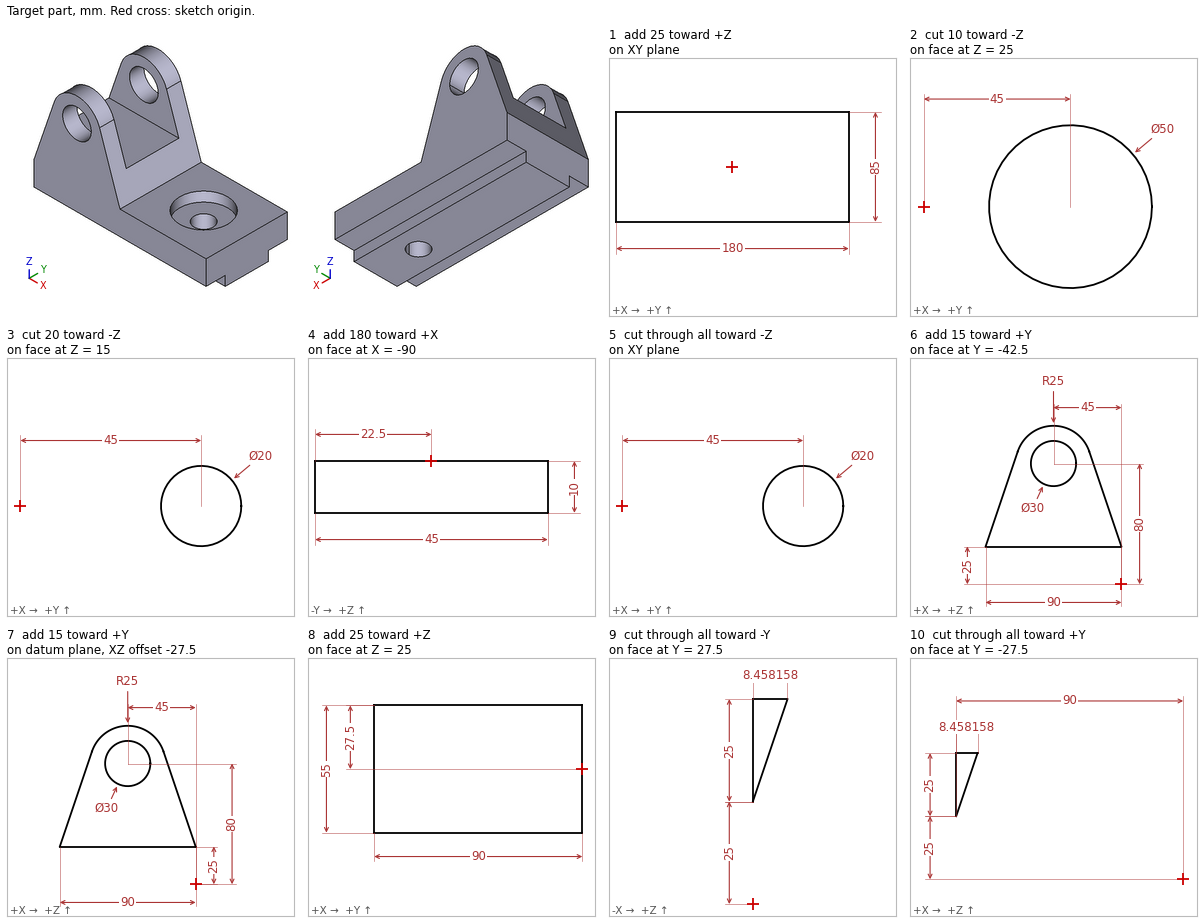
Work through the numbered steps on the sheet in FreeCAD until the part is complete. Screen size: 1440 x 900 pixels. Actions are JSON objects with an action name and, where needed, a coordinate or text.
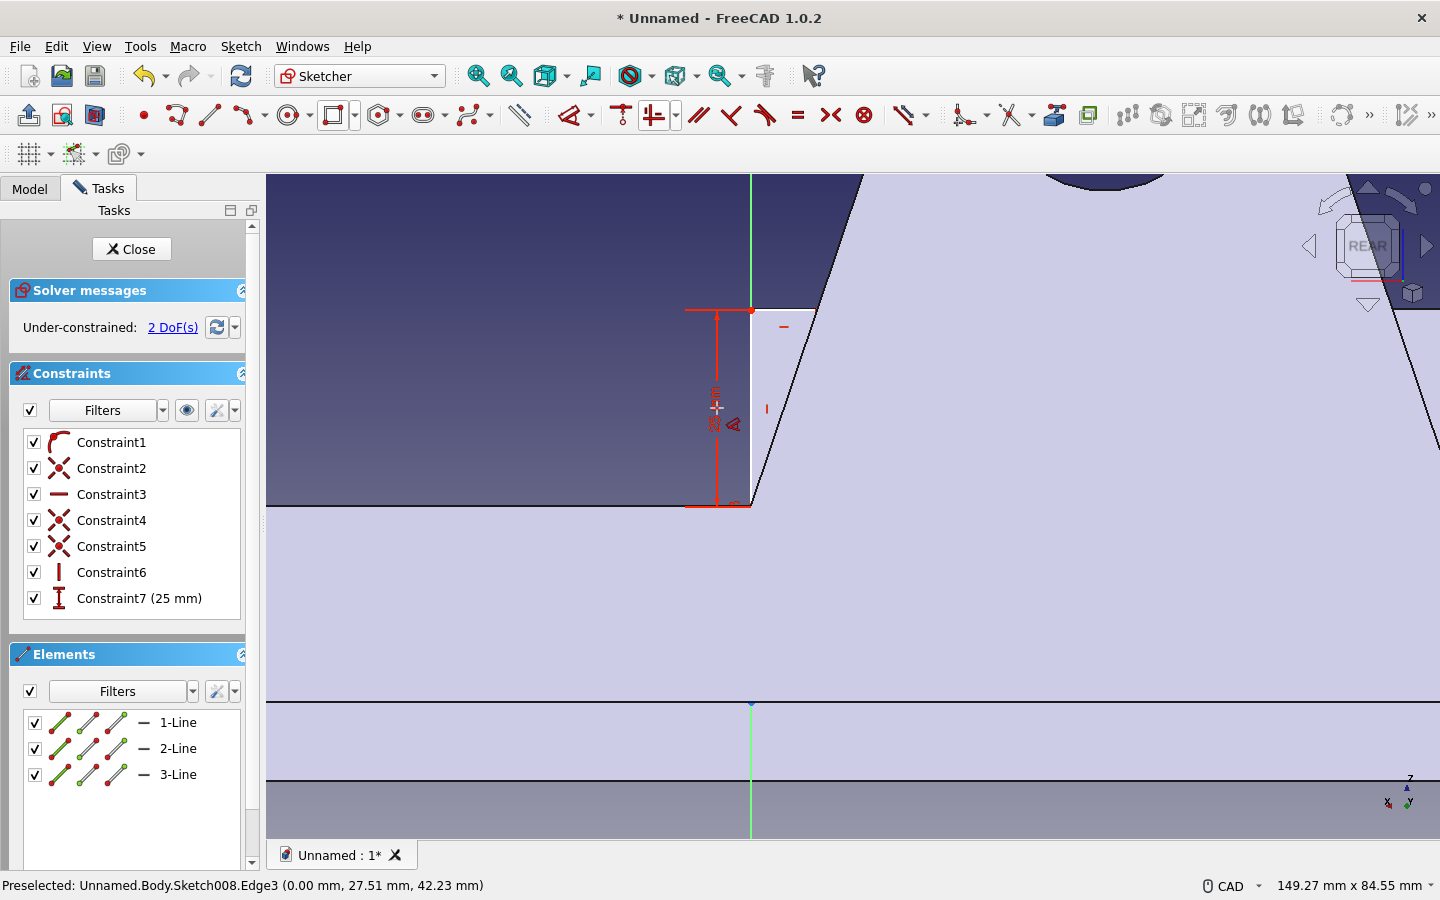
{"action": "left_click", "coordinate": [751, 507]}
{"action": "left_click", "coordinate": [717, 605]}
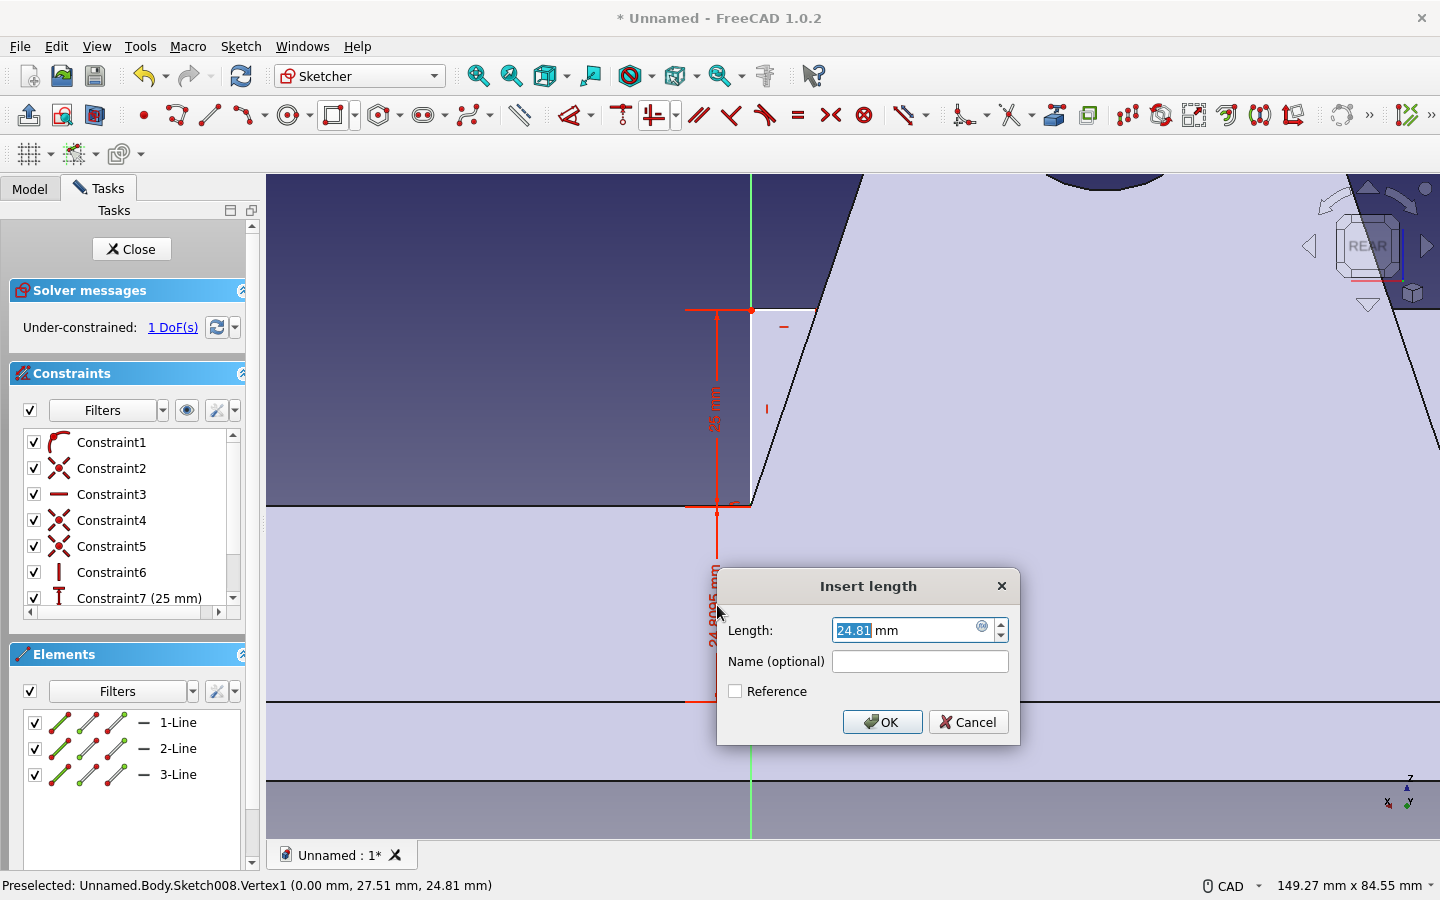
{"action": "type", "text": "25"}
{"action": "key", "text": "Return"}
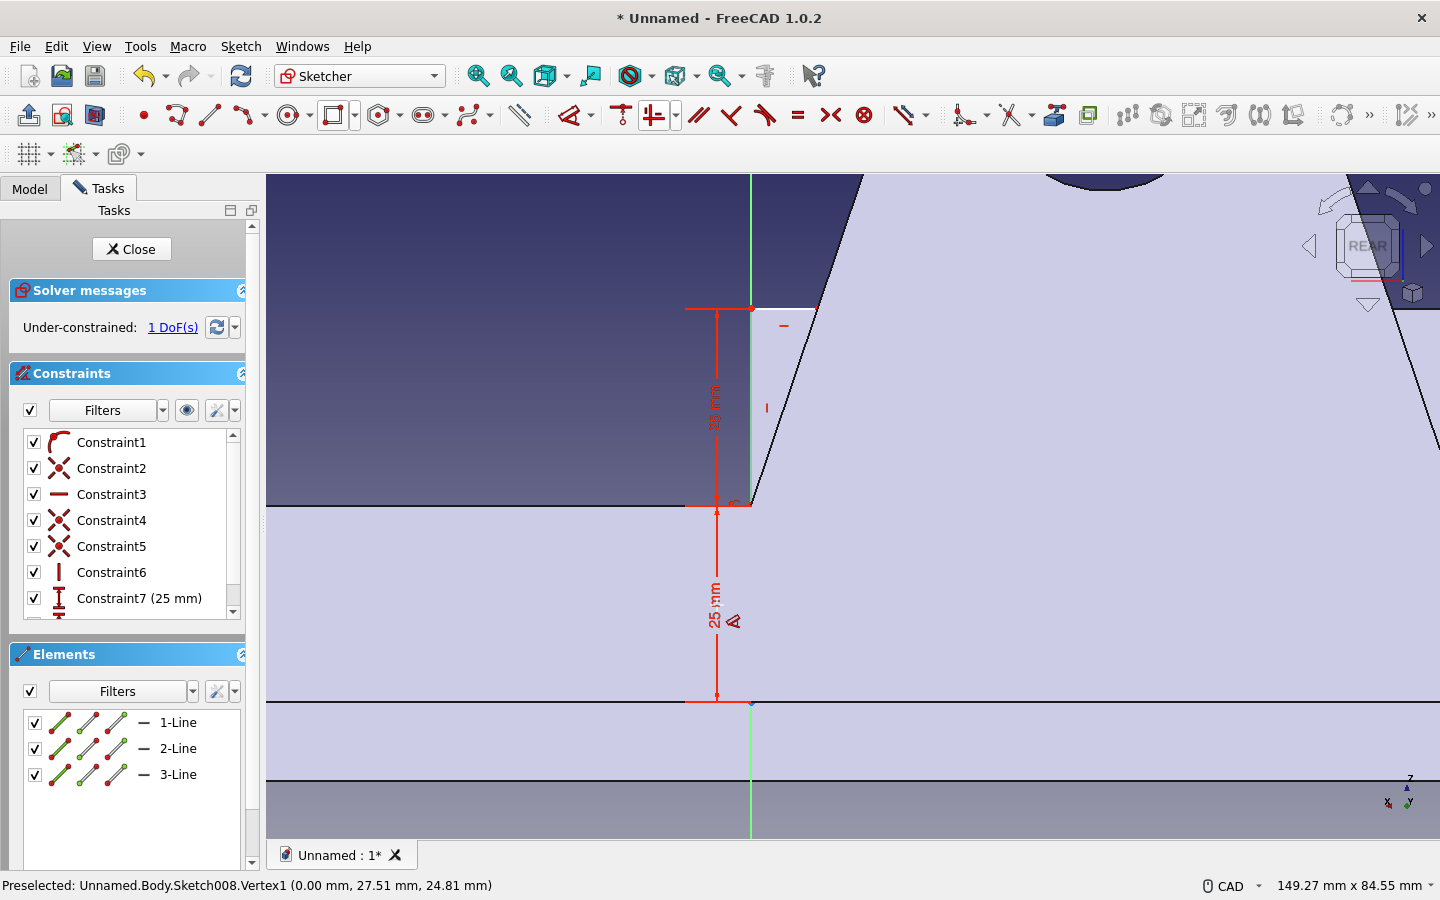
{"action": "left_click", "coordinate": [798, 309]}
{"action": "left_click", "coordinate": [785, 275]}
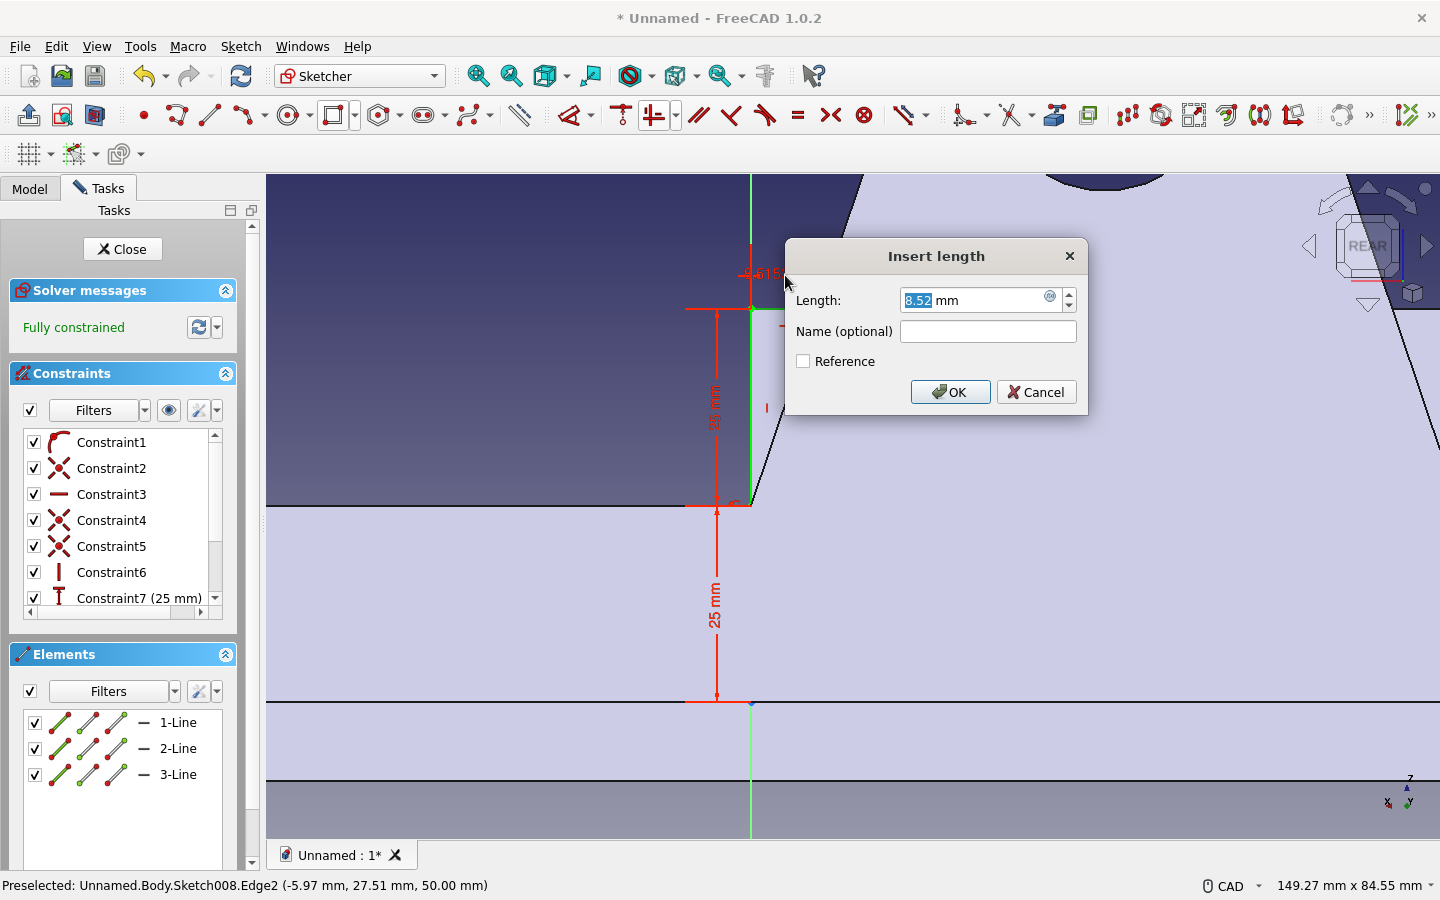
{"action": "type", "text": "8.458158"}
{"action": "key", "text": "Return"}
{"action": "key", "text": "Escape"}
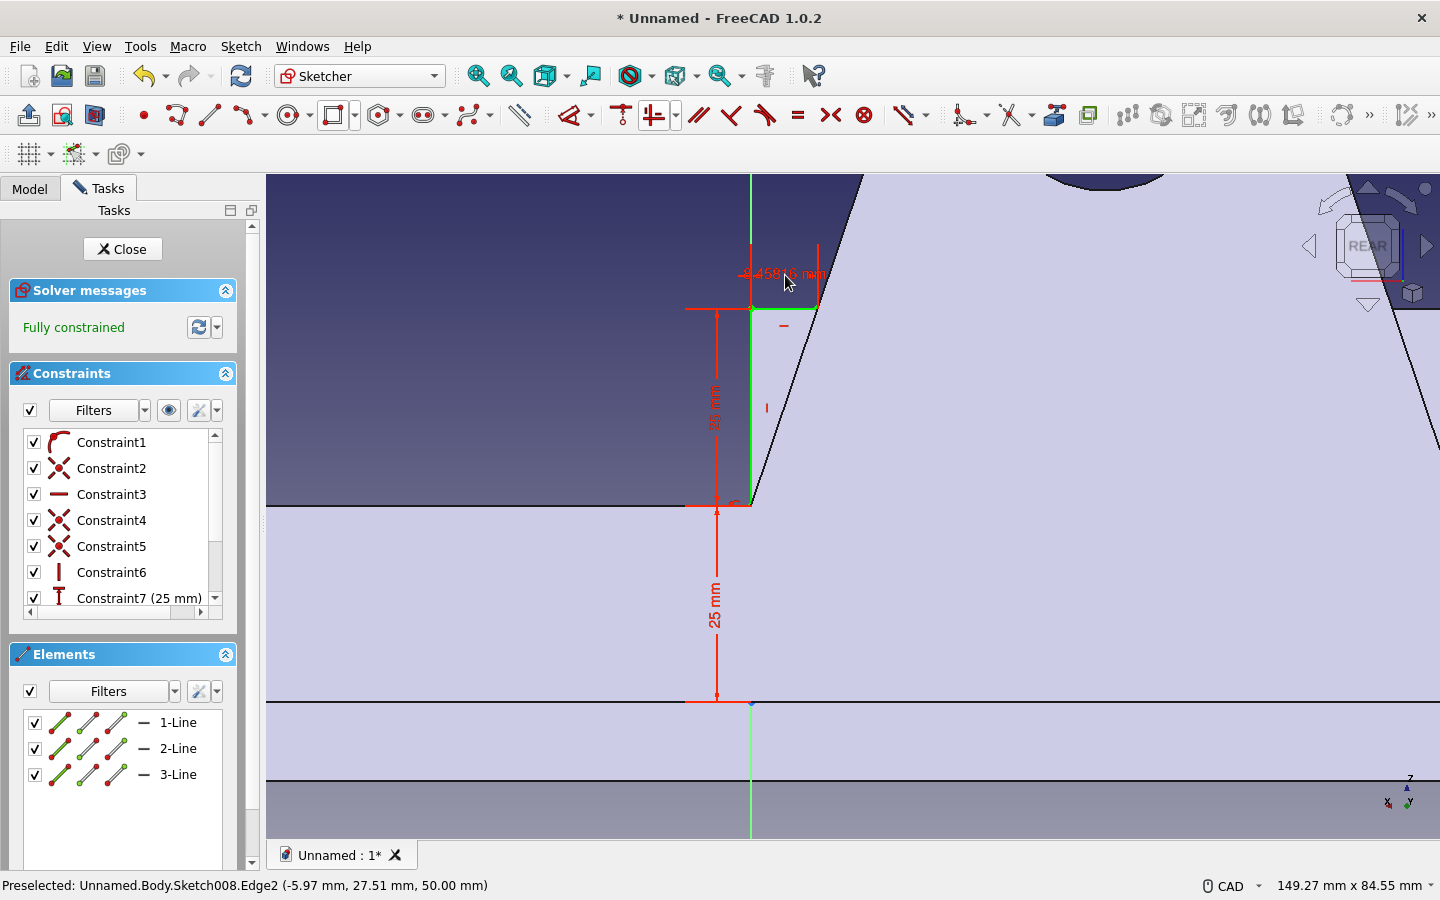
{"action": "left_click", "coordinate": [123, 249]}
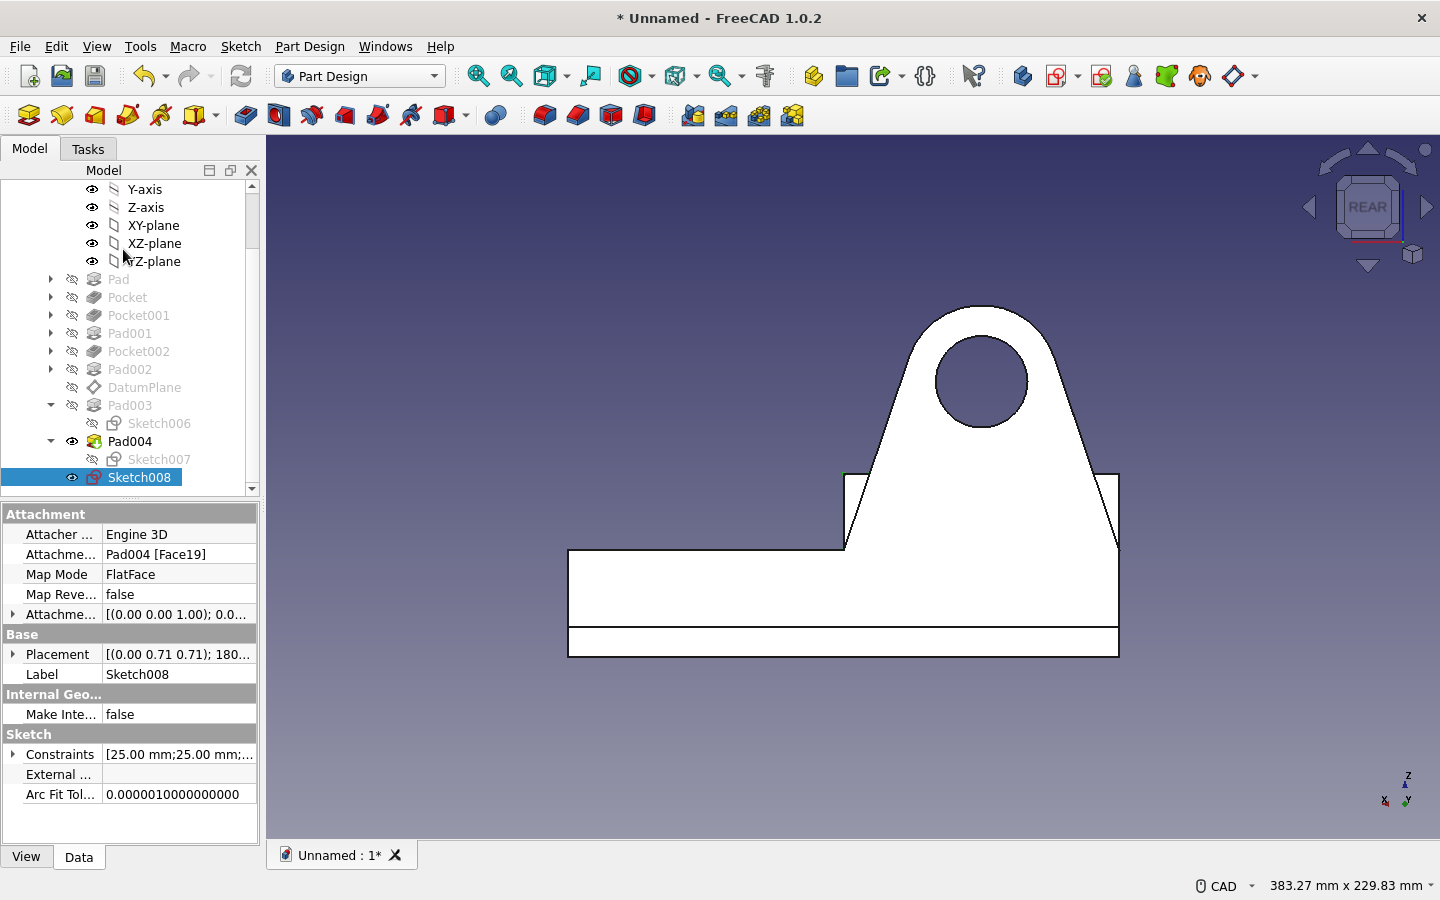
{"action": "left_click", "coordinate": [246, 116]}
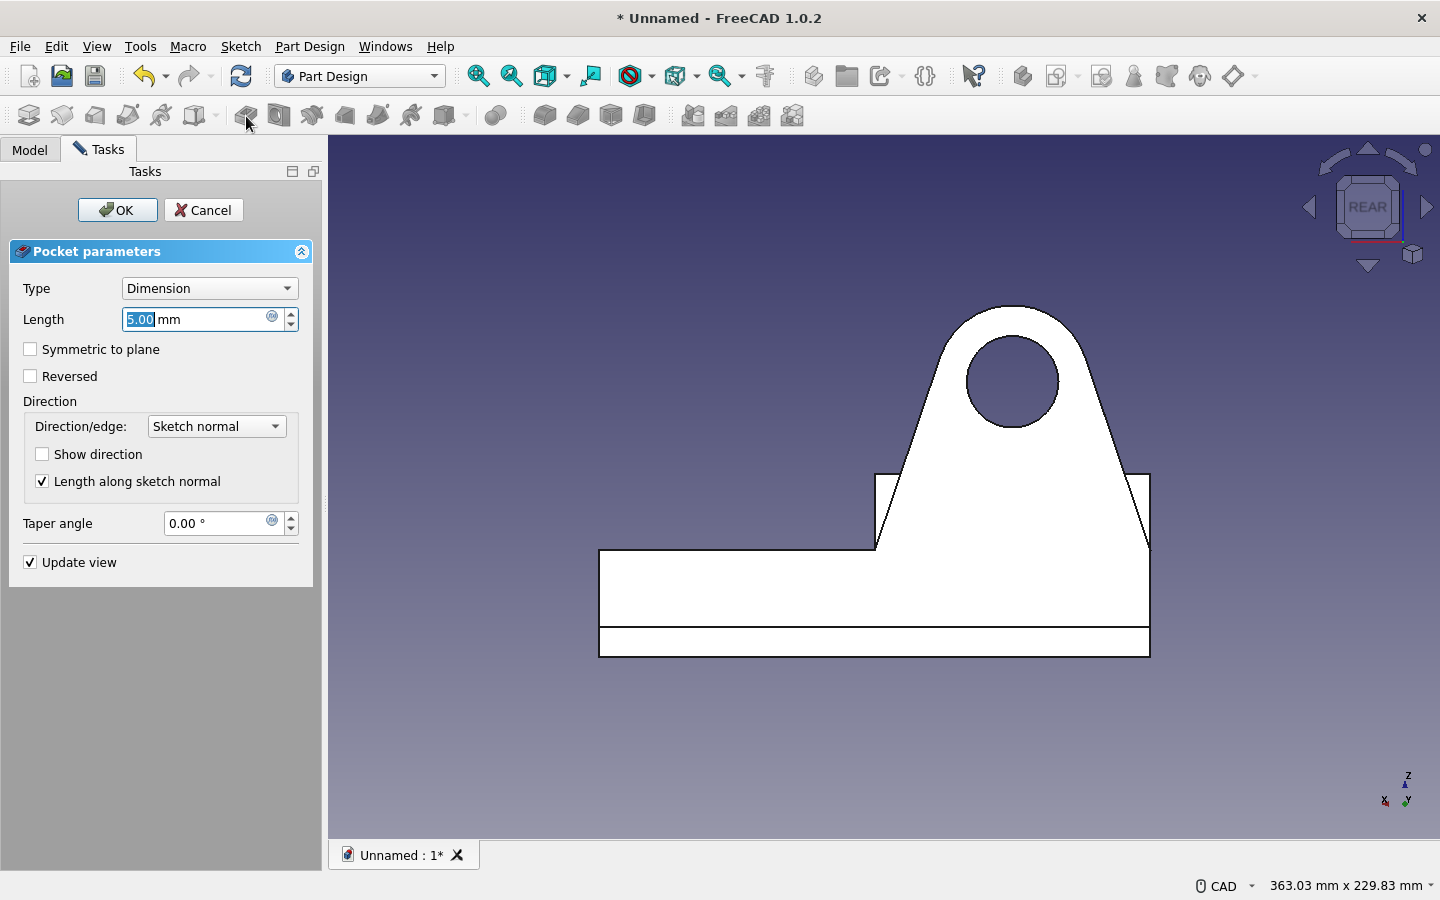
{"action": "left_click", "coordinate": [210, 288]}